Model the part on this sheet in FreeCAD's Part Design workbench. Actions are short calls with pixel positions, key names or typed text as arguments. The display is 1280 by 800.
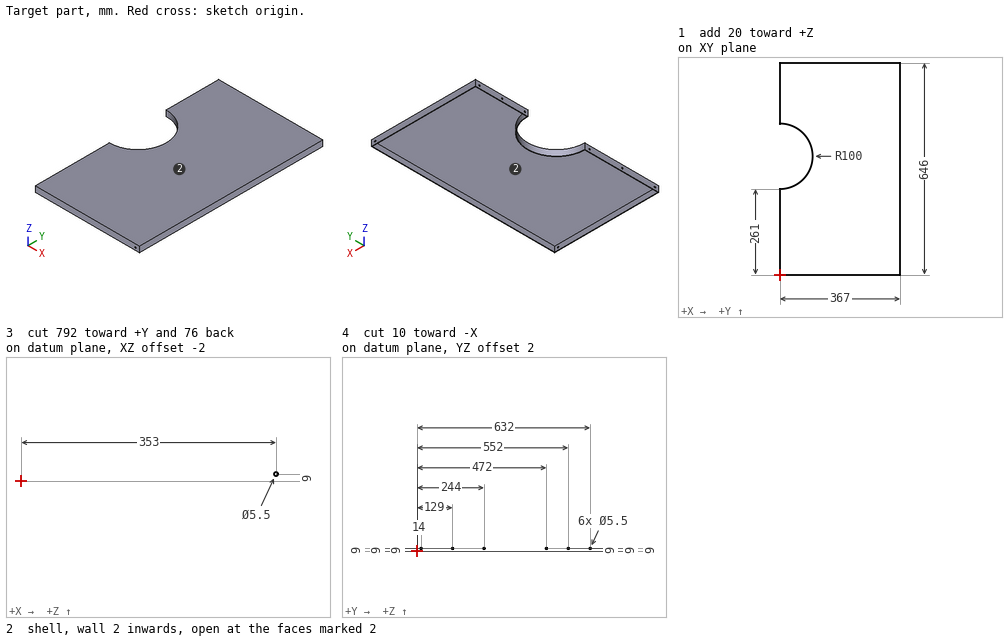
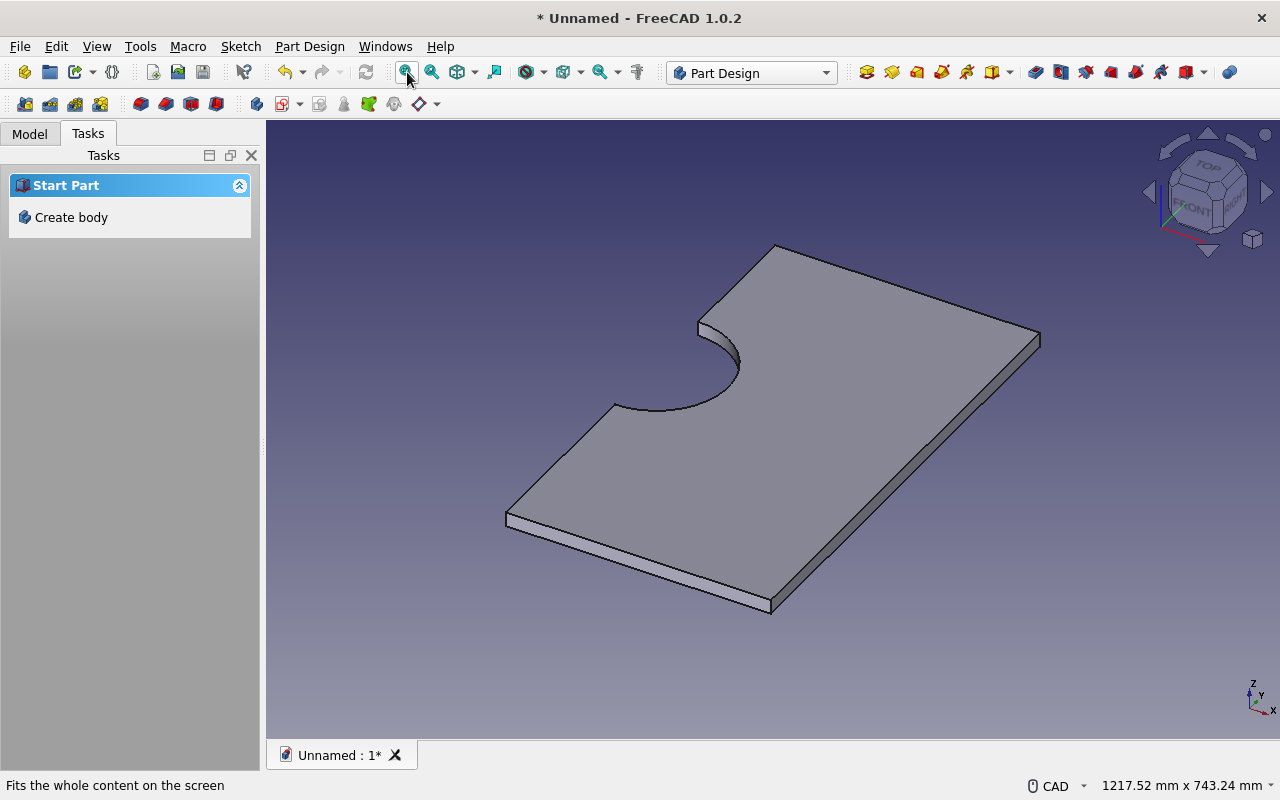
key(0)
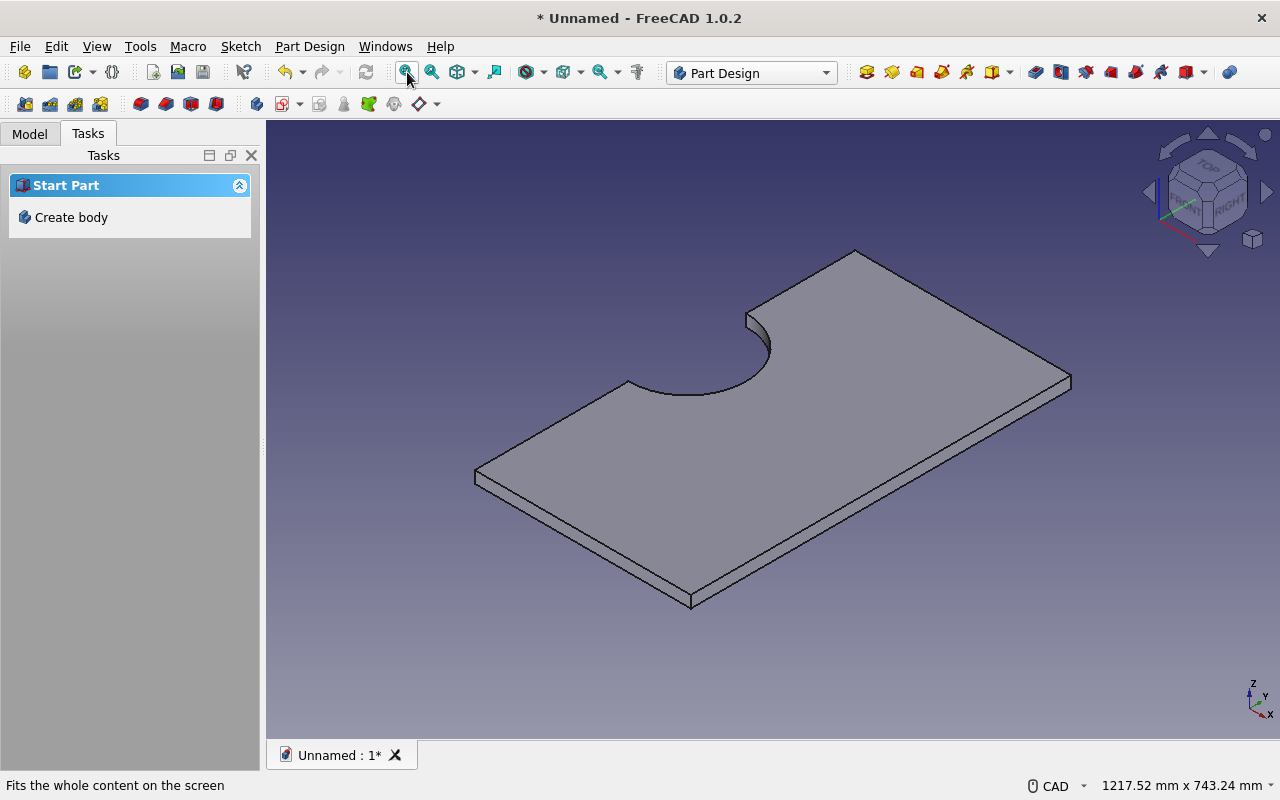
key(2)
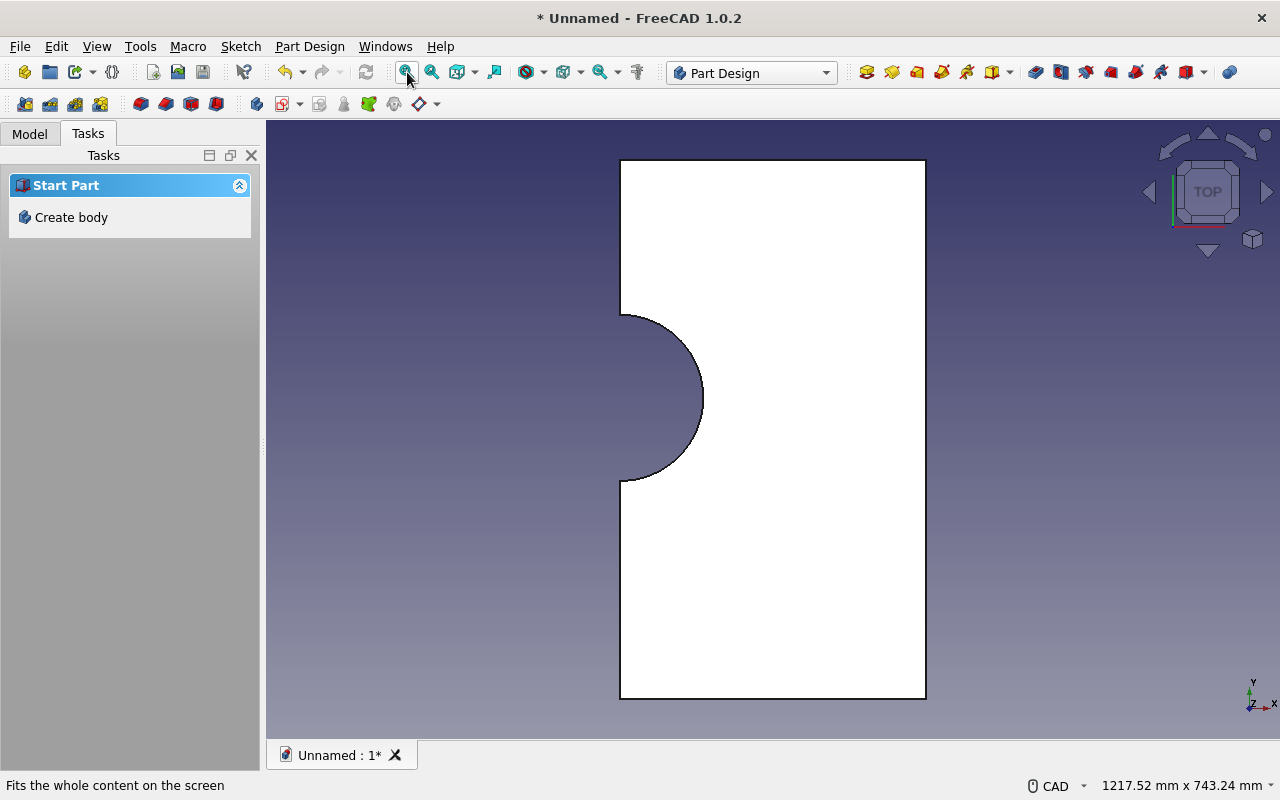
key(1)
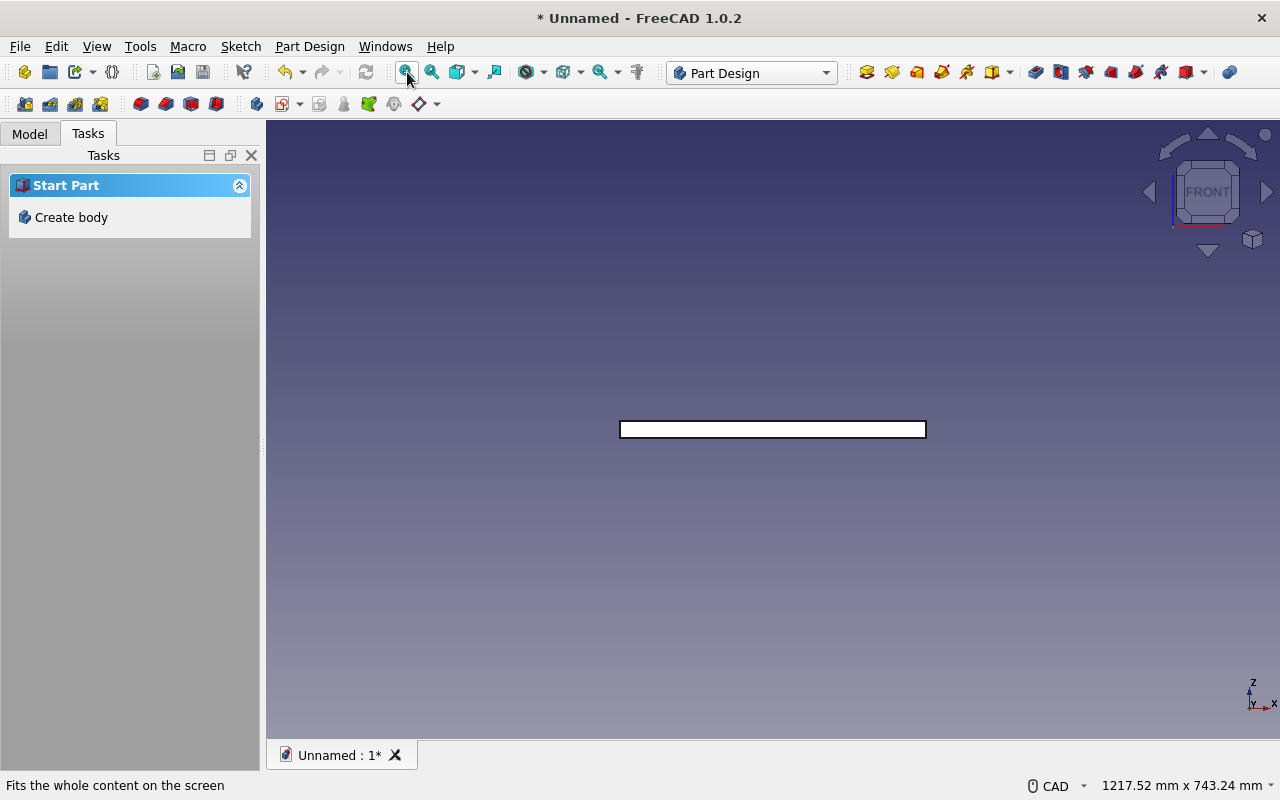
click(407, 72)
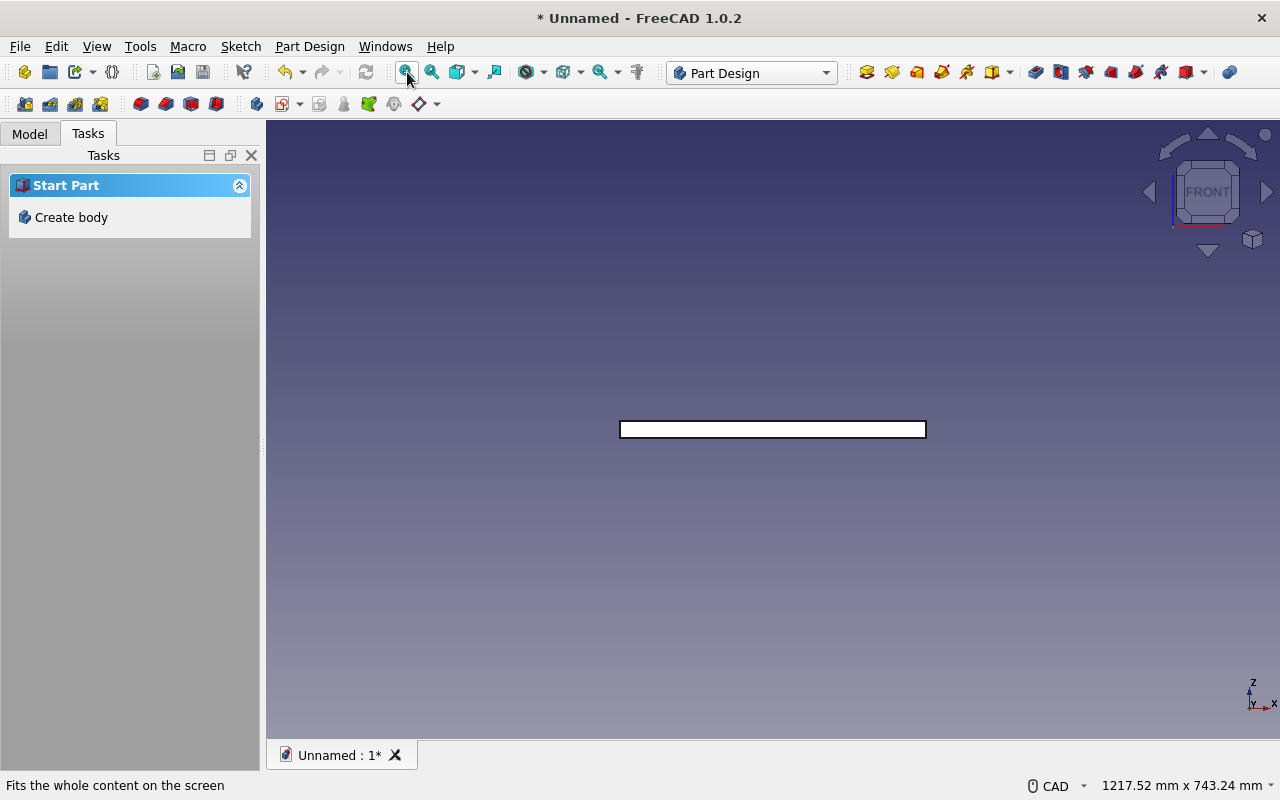
key(3)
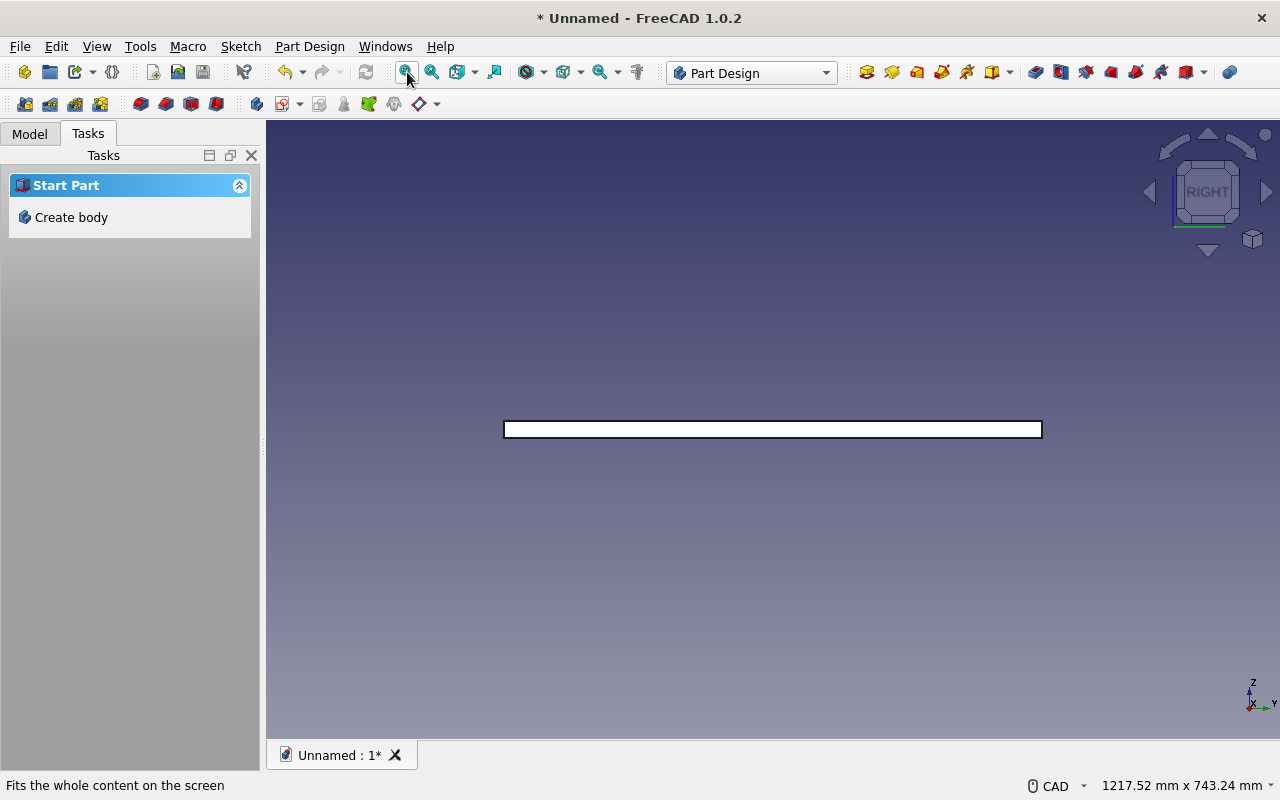
key(5)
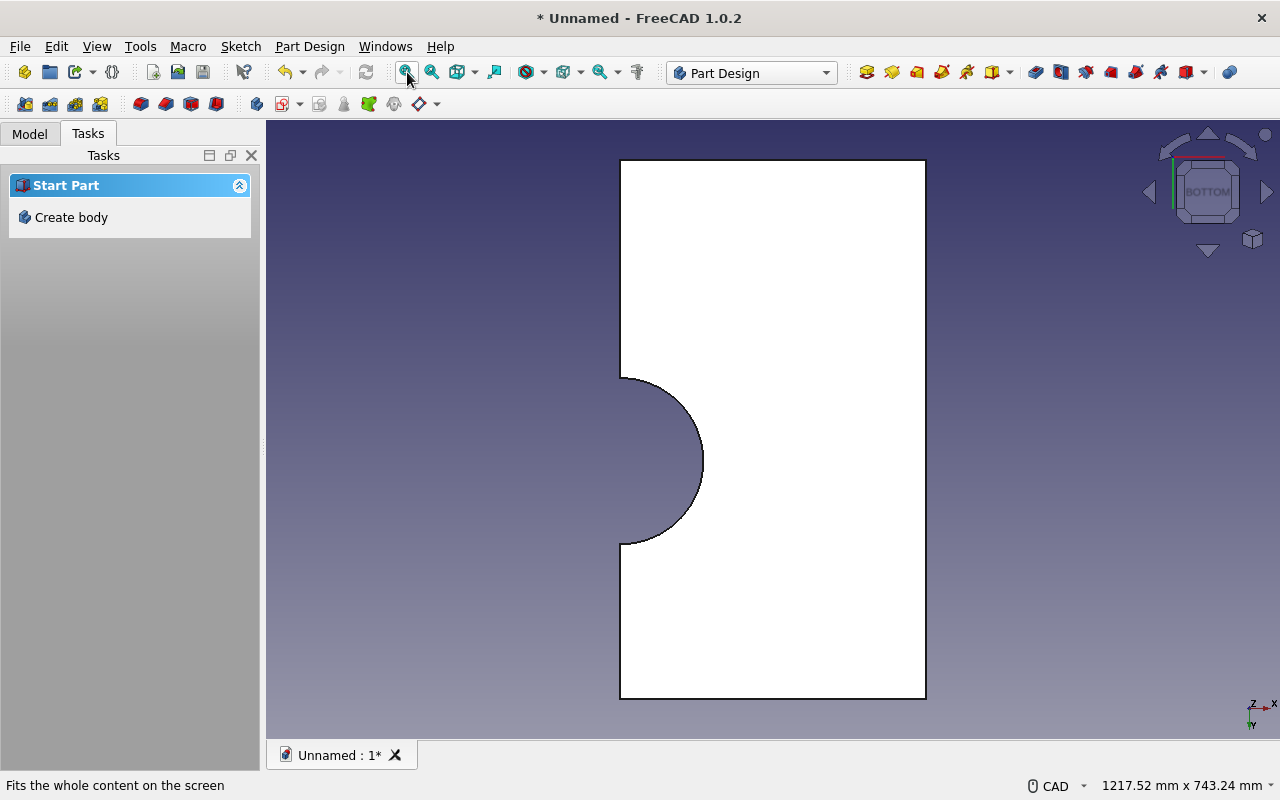
click(773, 275)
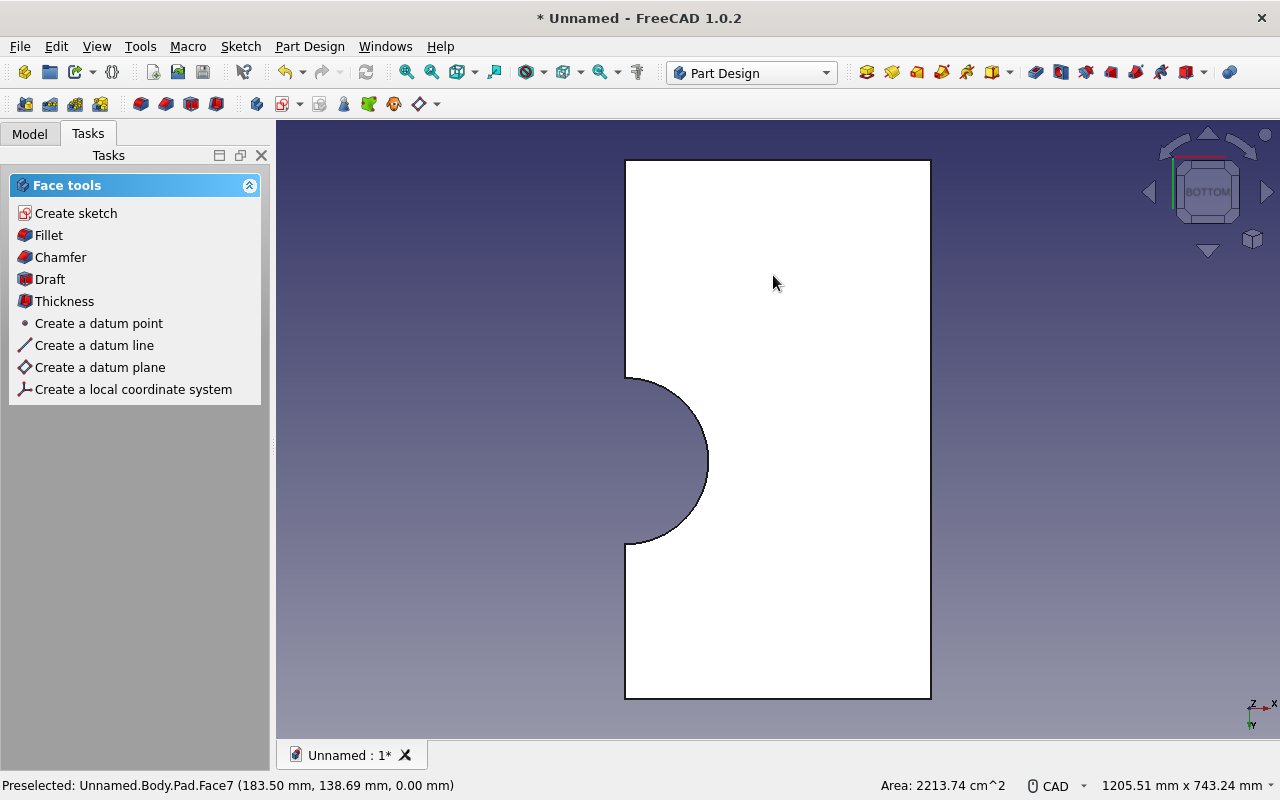
click(216, 104)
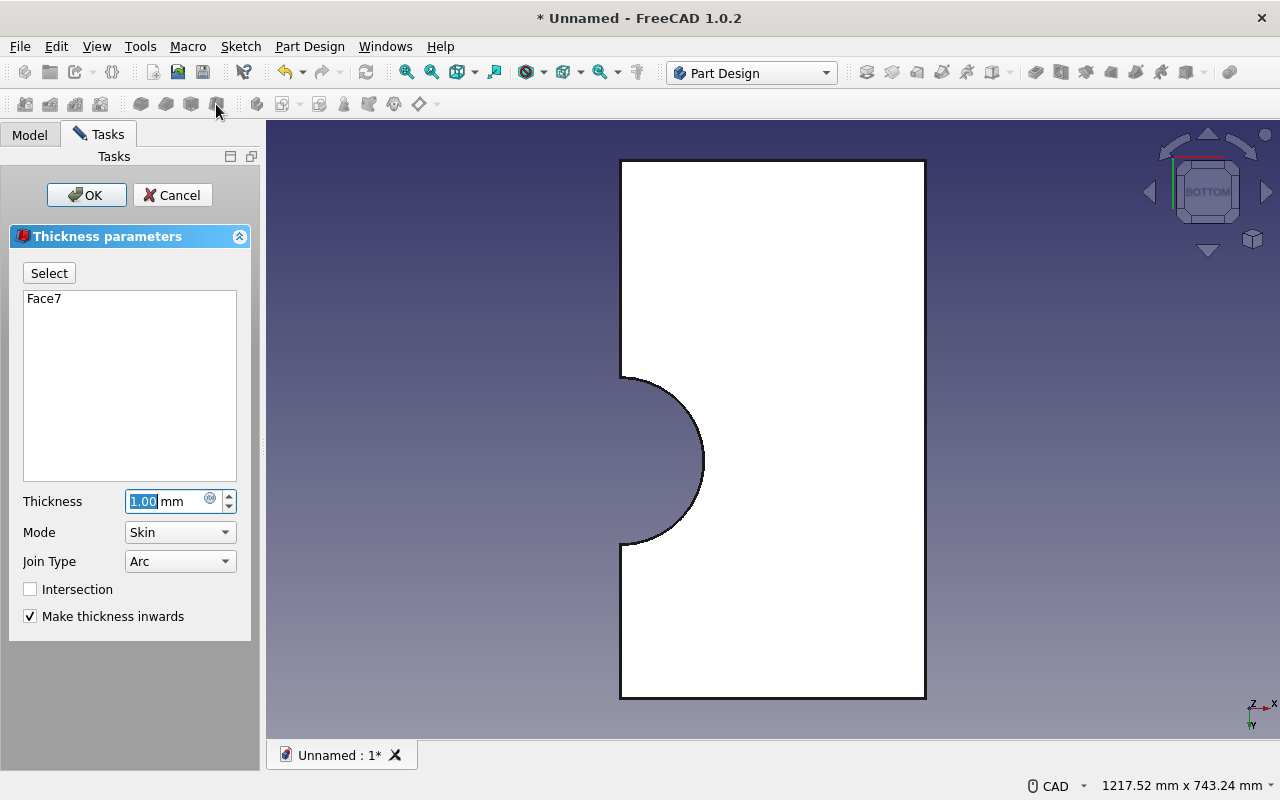
text(2)
key(Tab)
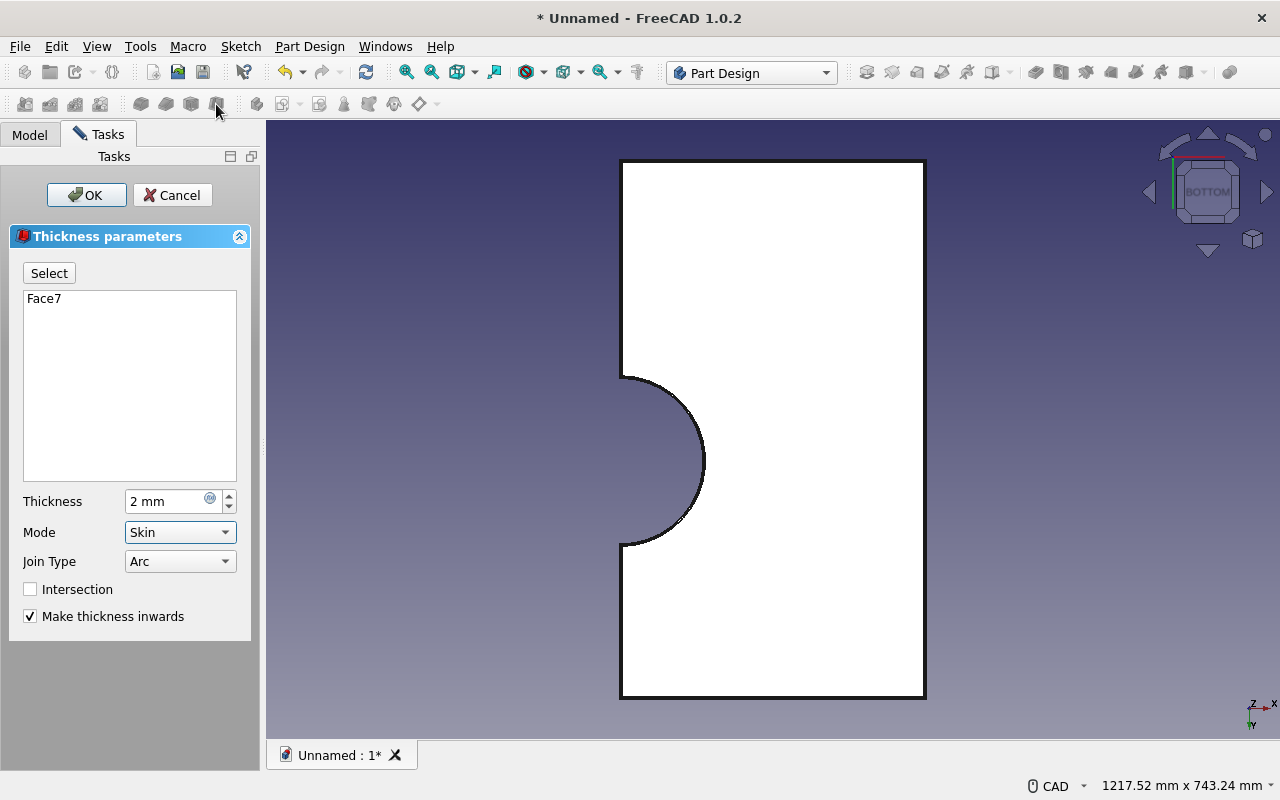
click(181, 562)